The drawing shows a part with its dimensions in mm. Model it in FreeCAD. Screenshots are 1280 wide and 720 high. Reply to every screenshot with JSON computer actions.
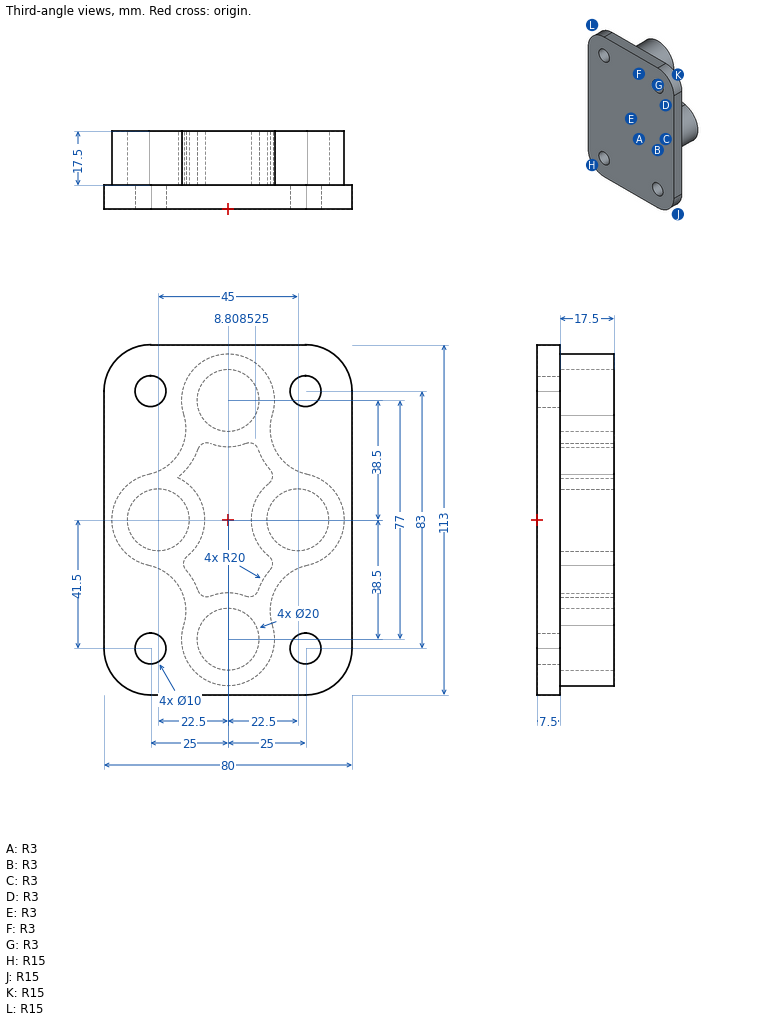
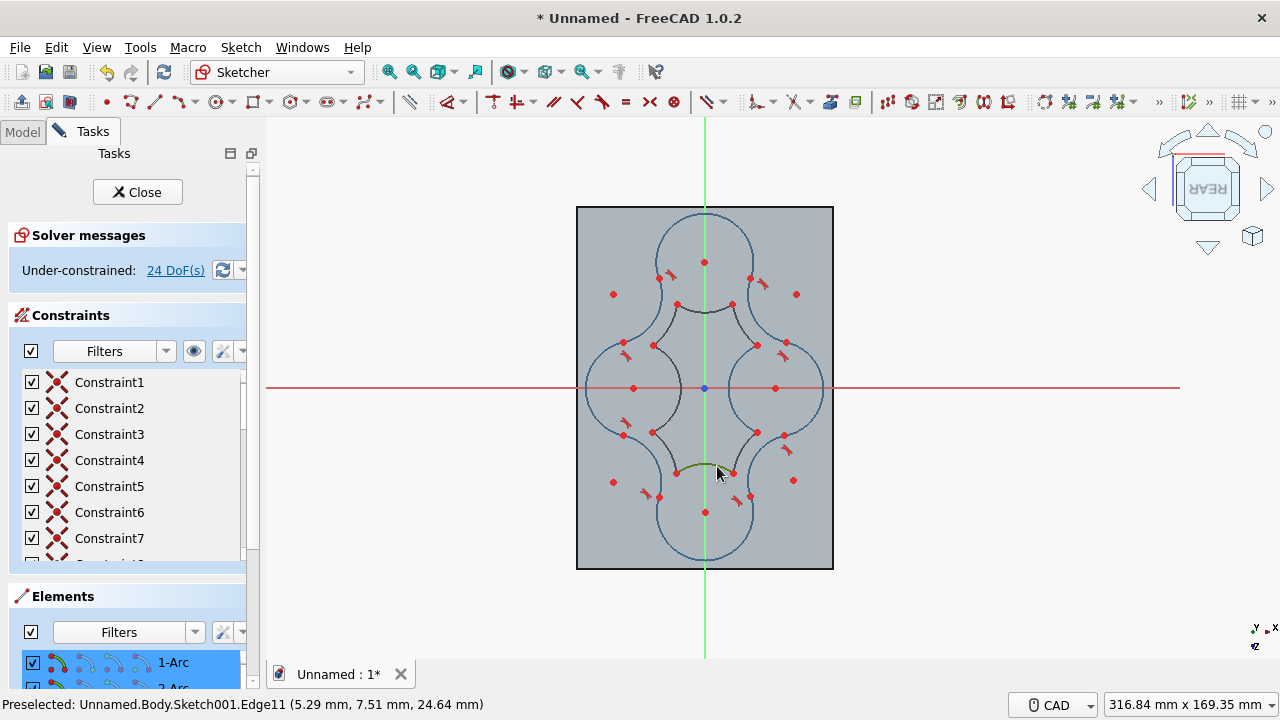
{"action": "left_click", "coordinate": [676, 410]}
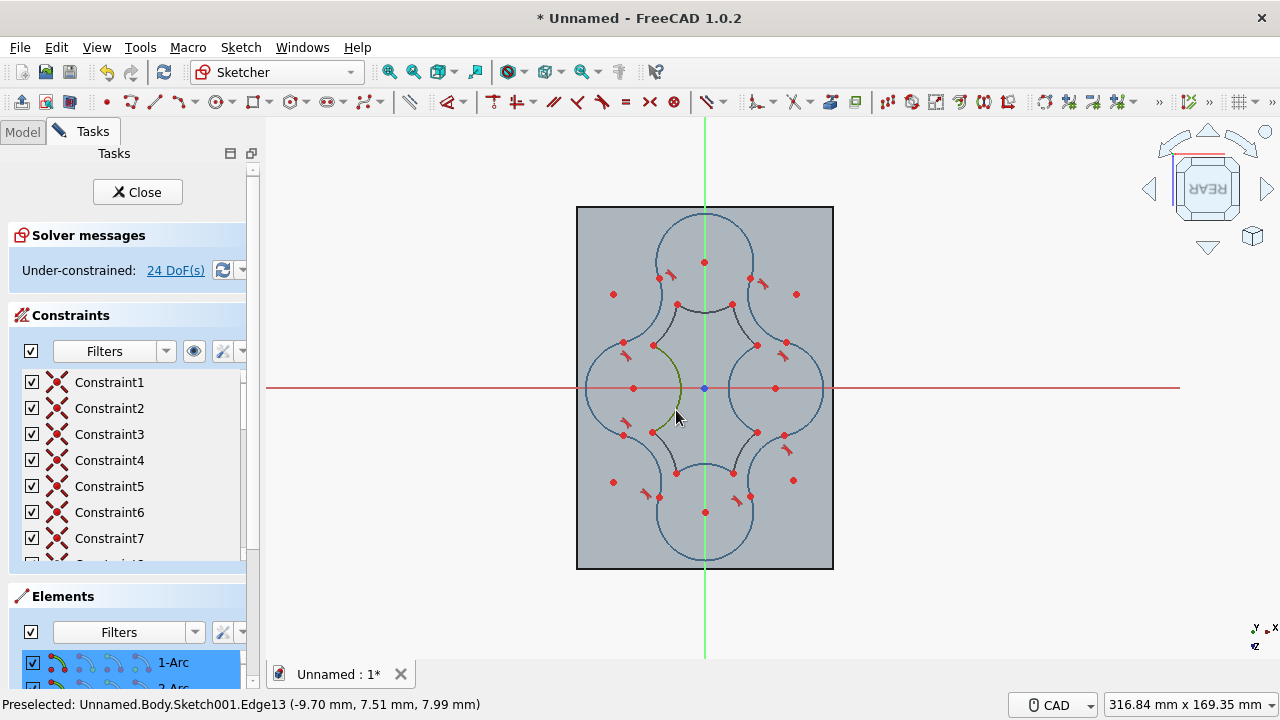
{"action": "left_click", "coordinate": [693, 311]}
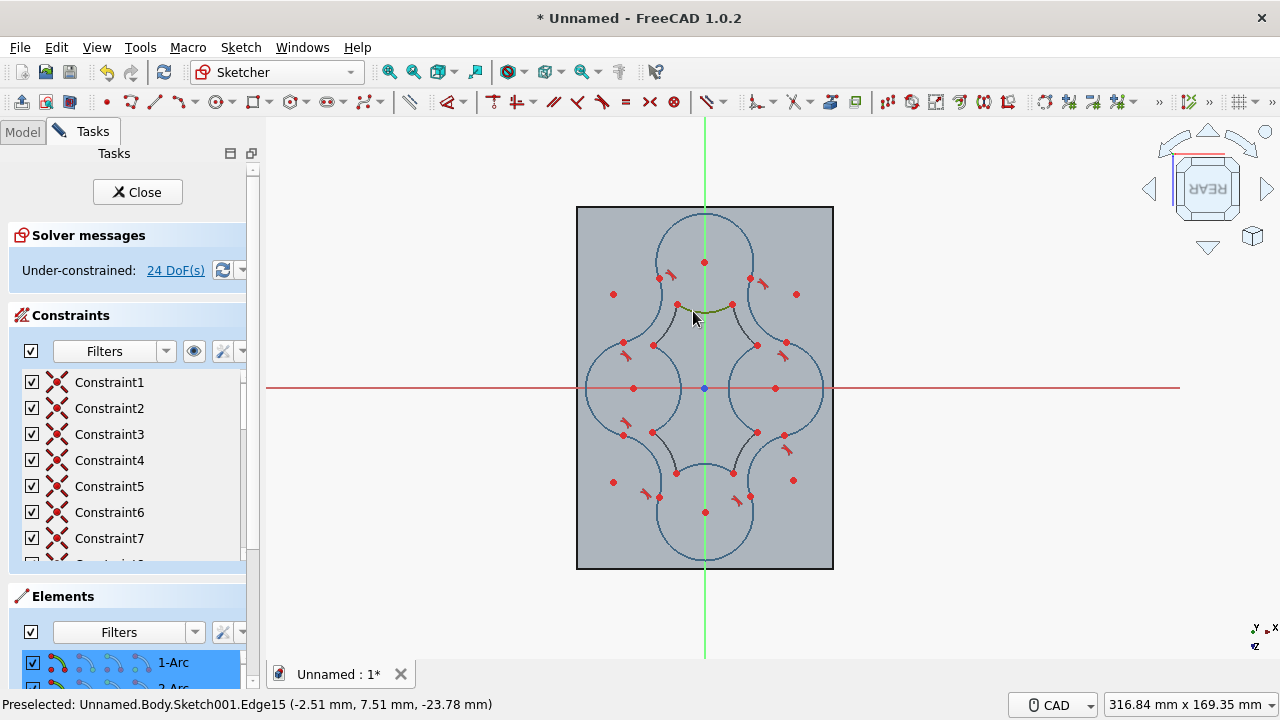
{"action": "key", "text": "e"}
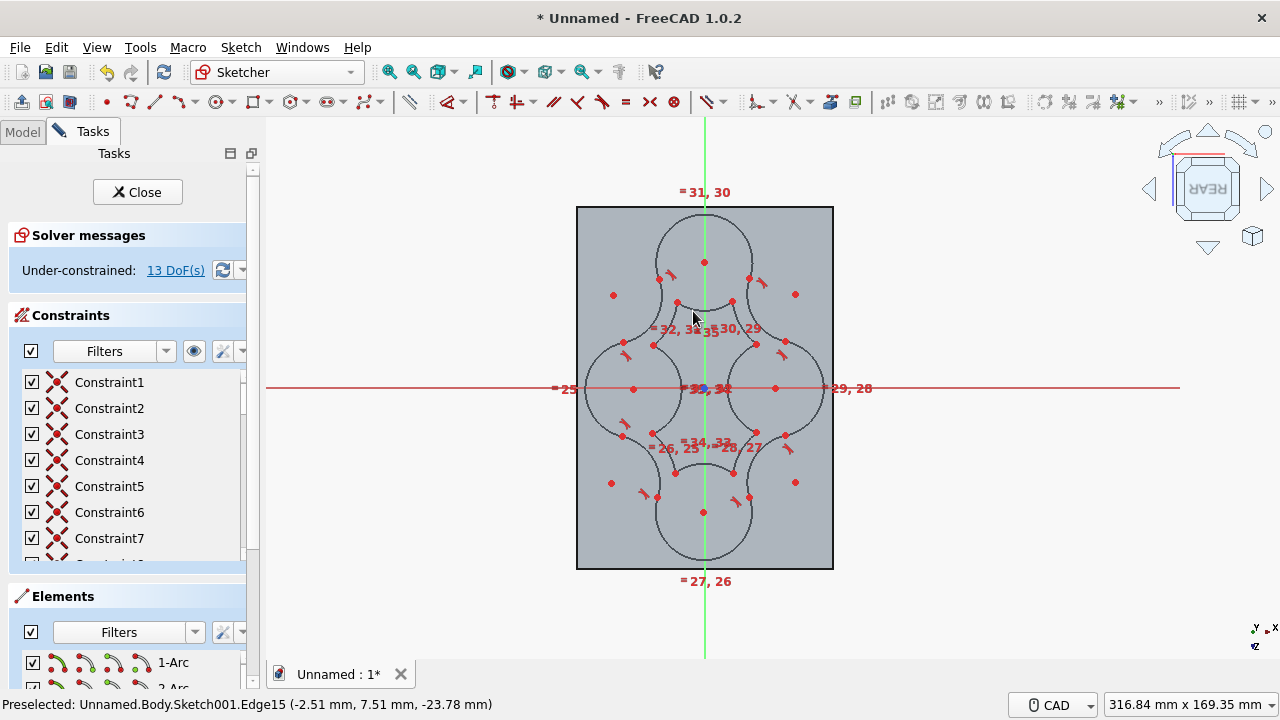
{"action": "left_click", "coordinate": [737, 460]}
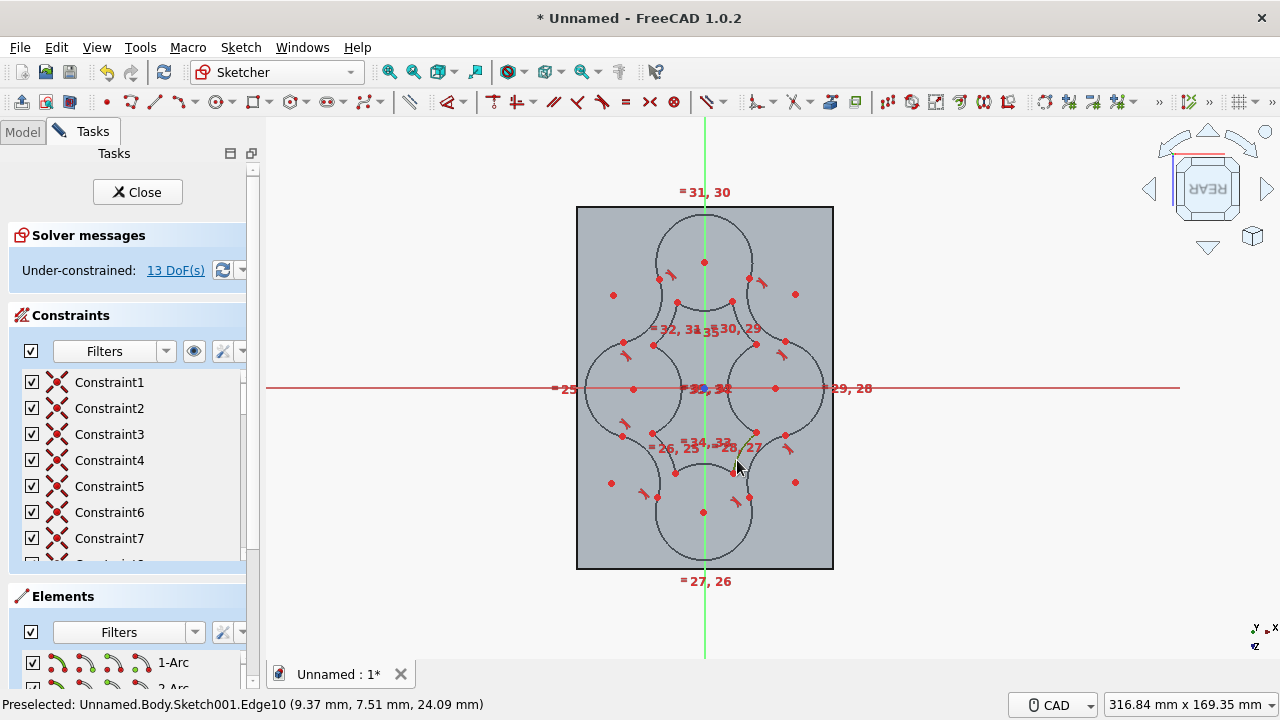
{"action": "left_click", "coordinate": [672, 460]}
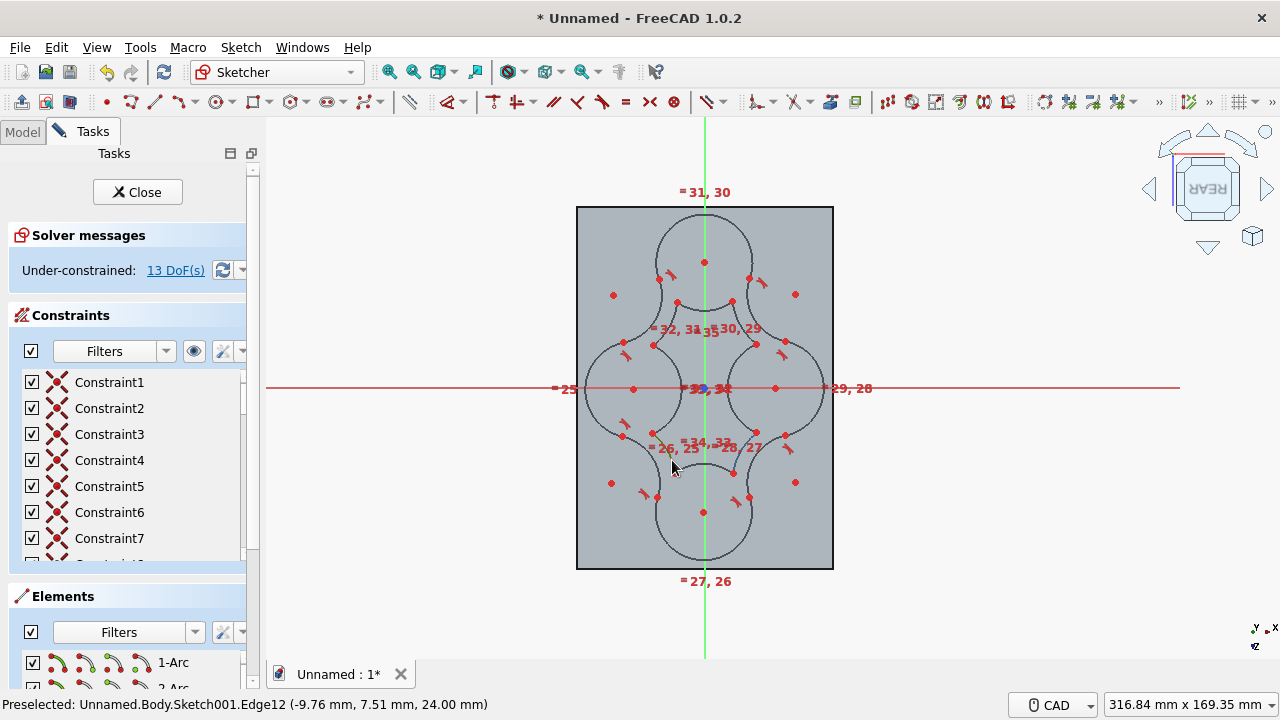
{"action": "left_click", "coordinate": [674, 317]}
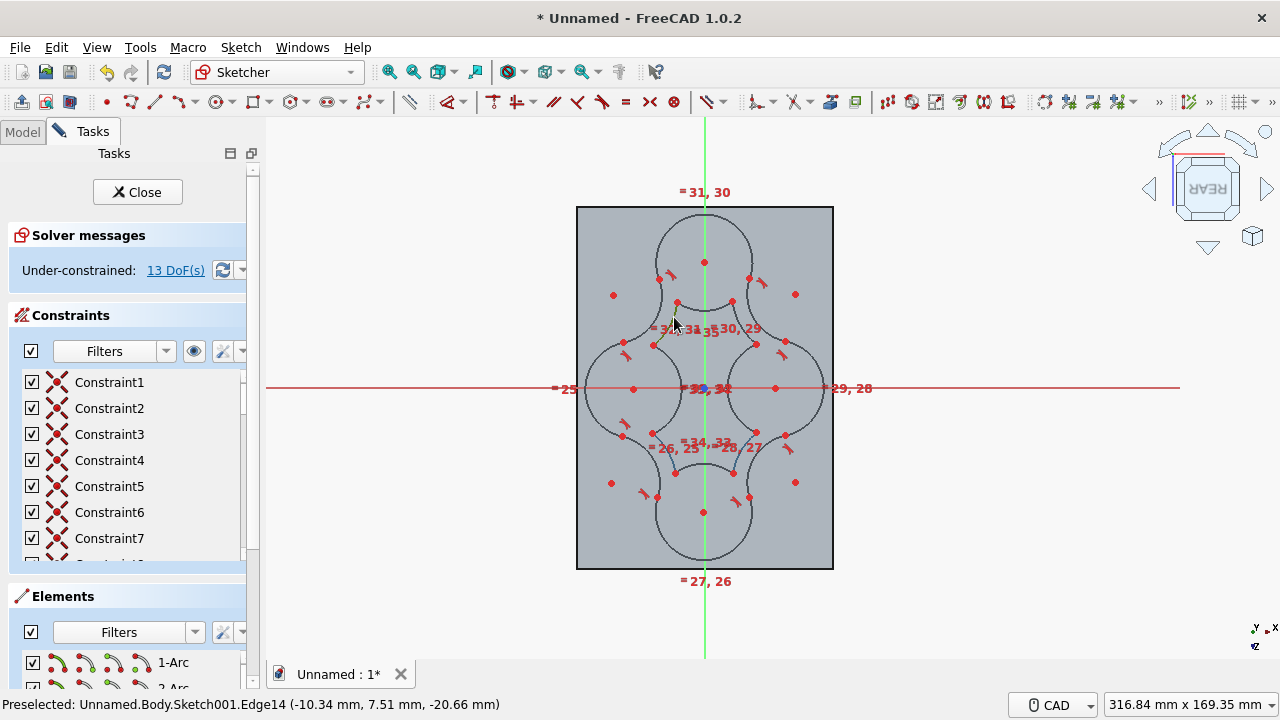
{"action": "left_click", "coordinate": [736, 316]}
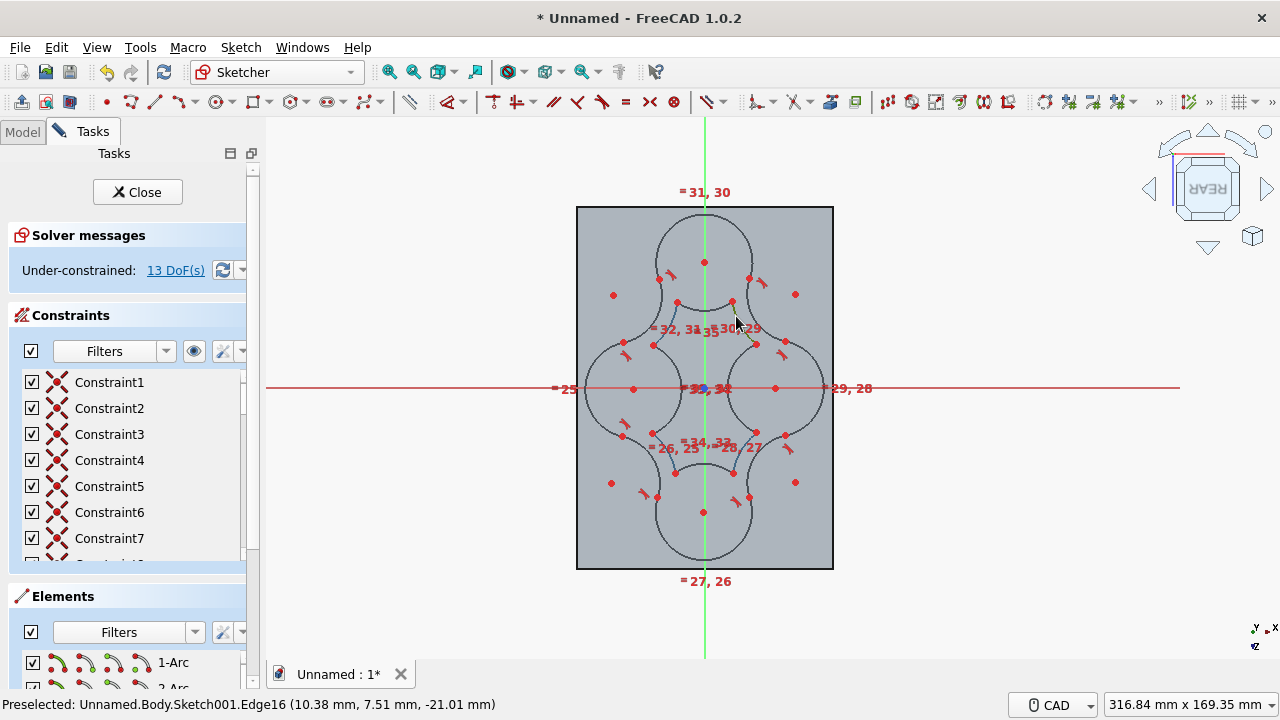
{"action": "left_click", "coordinate": [626, 102]}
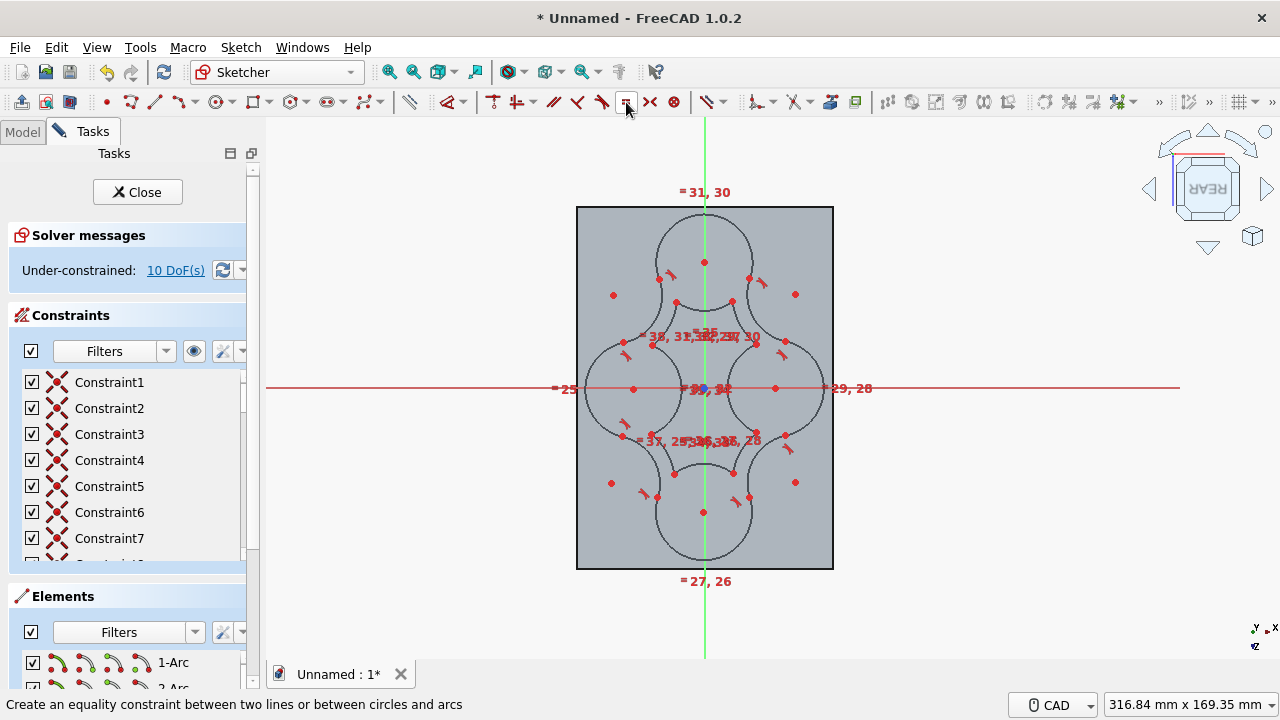
{"action": "left_click", "coordinate": [633, 390]}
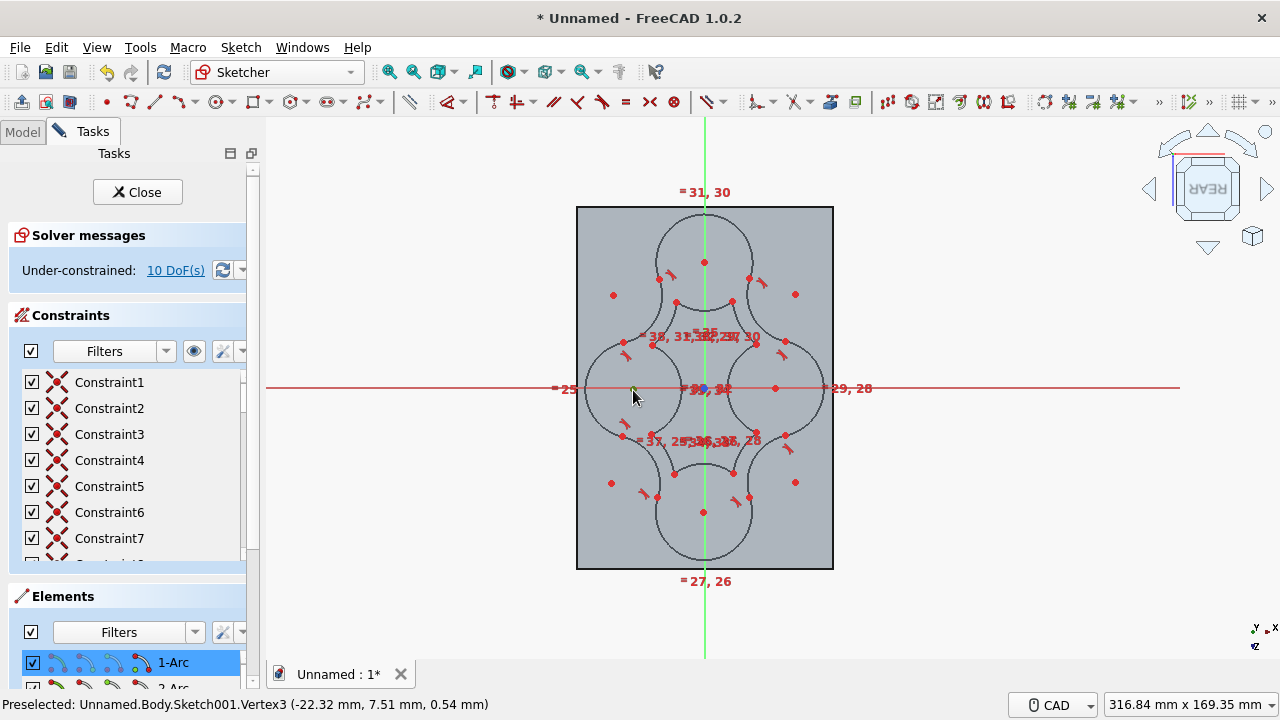
{"action": "left_click", "coordinate": [353, 388]}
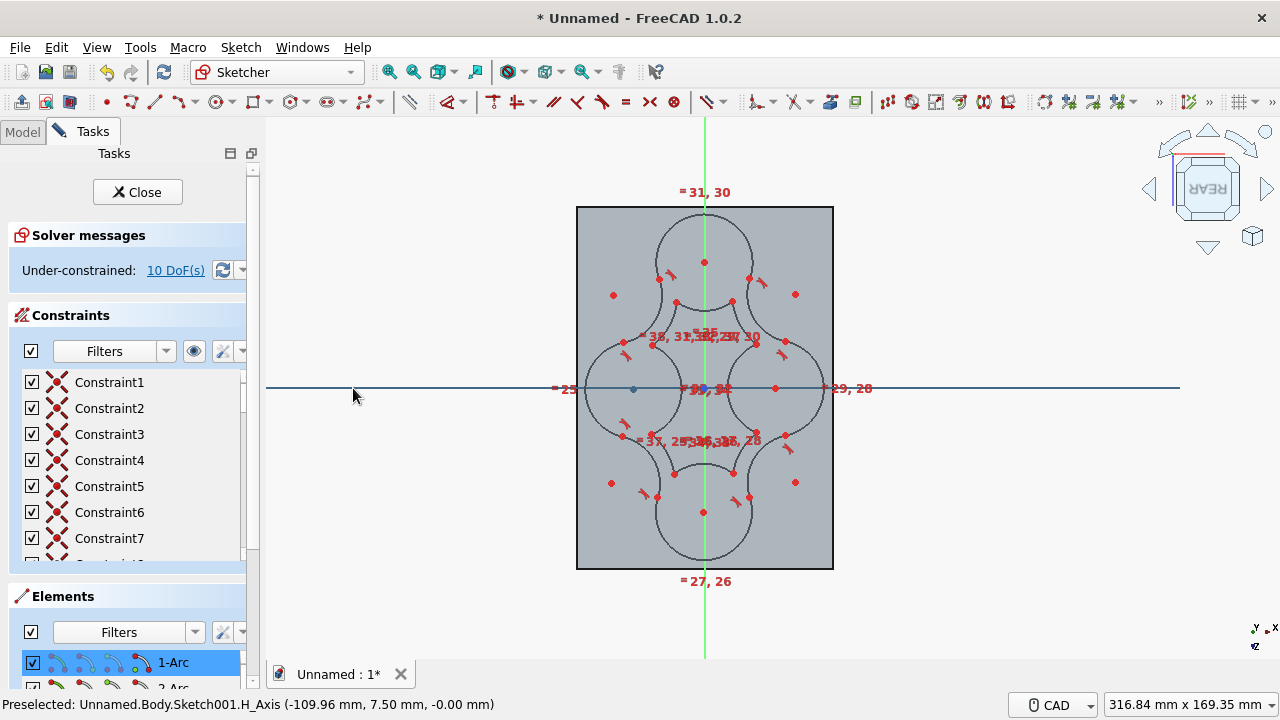
{"action": "key", "text": "c"}